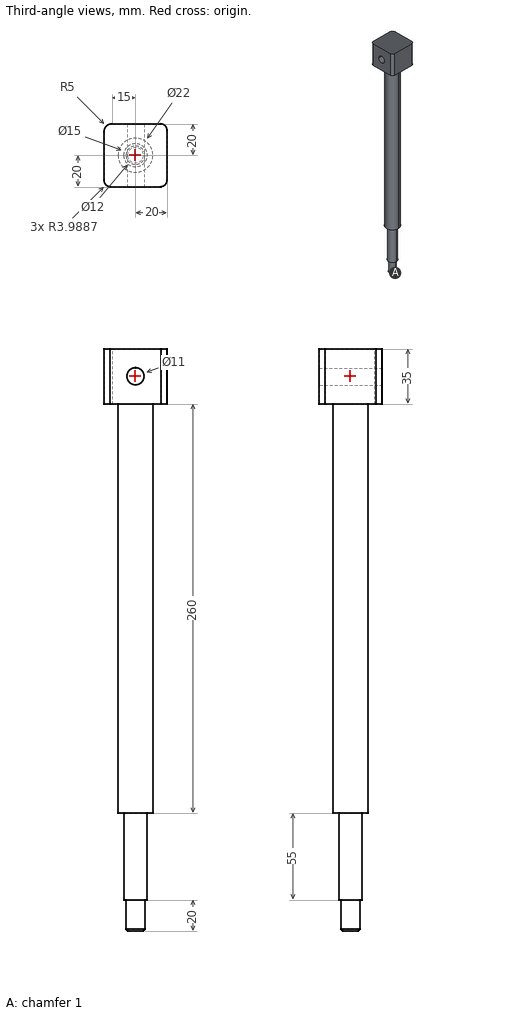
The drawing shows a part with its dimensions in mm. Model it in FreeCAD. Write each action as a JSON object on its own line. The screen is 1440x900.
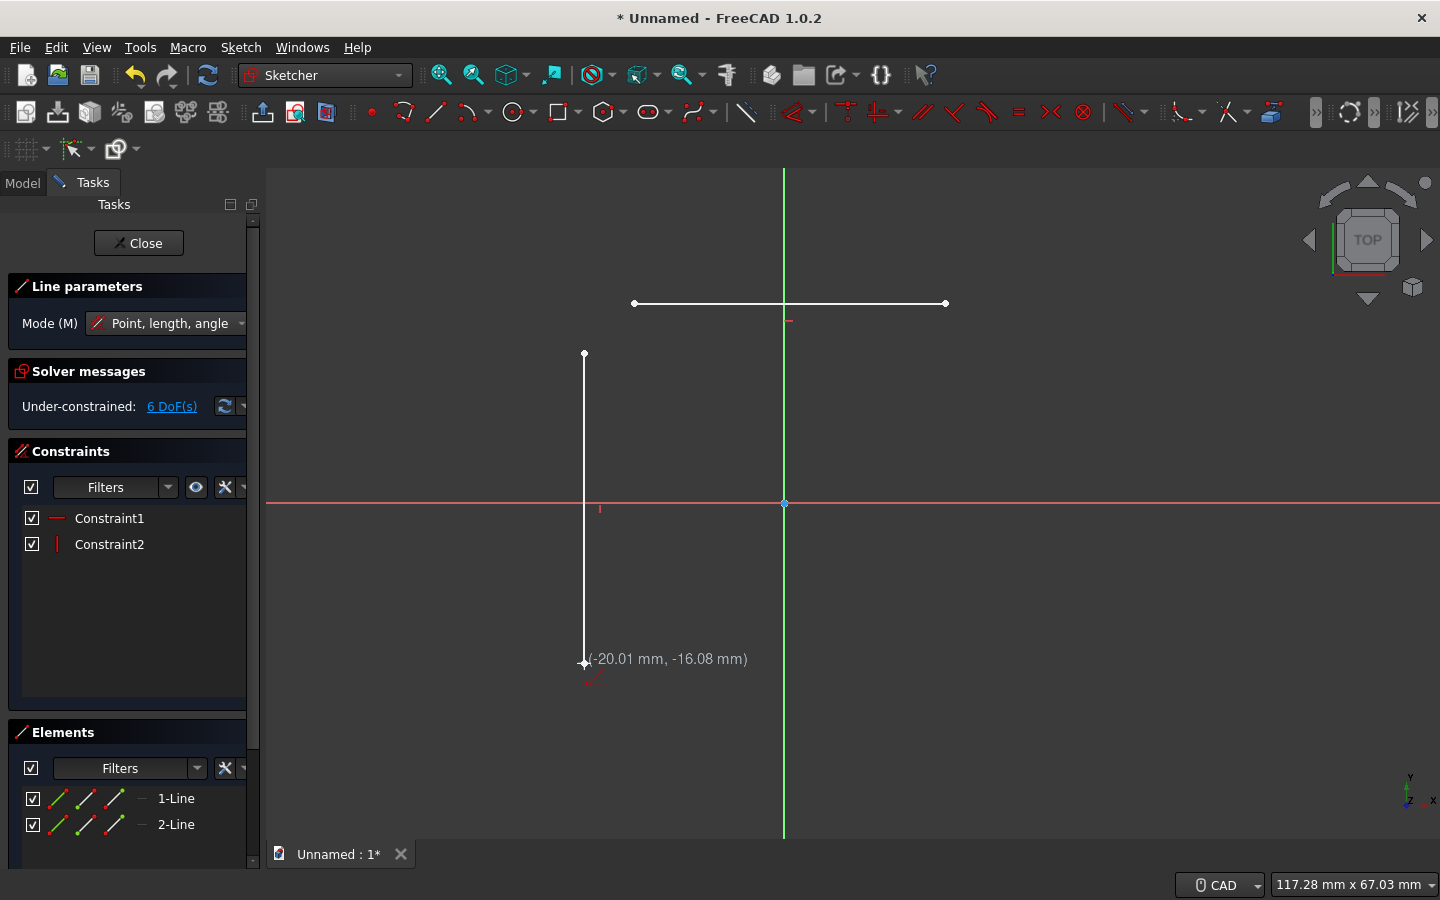
{"action": "left_click", "coordinate": [624, 703]}
{"action": "left_click", "coordinate": [945, 703]}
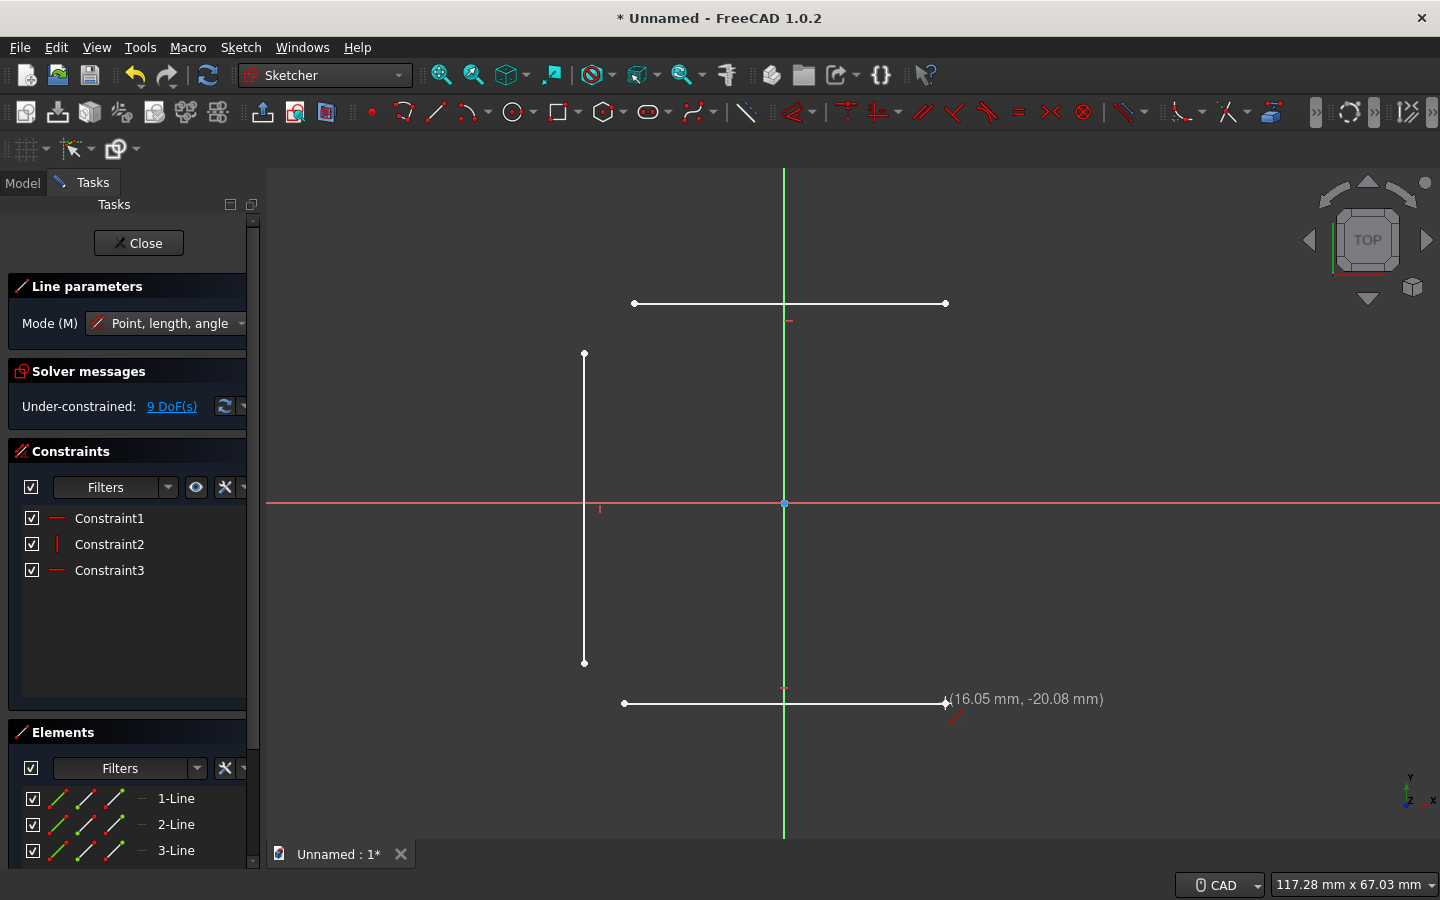
{"action": "left_click", "coordinate": [985, 663]}
{"action": "left_click", "coordinate": [985, 343]}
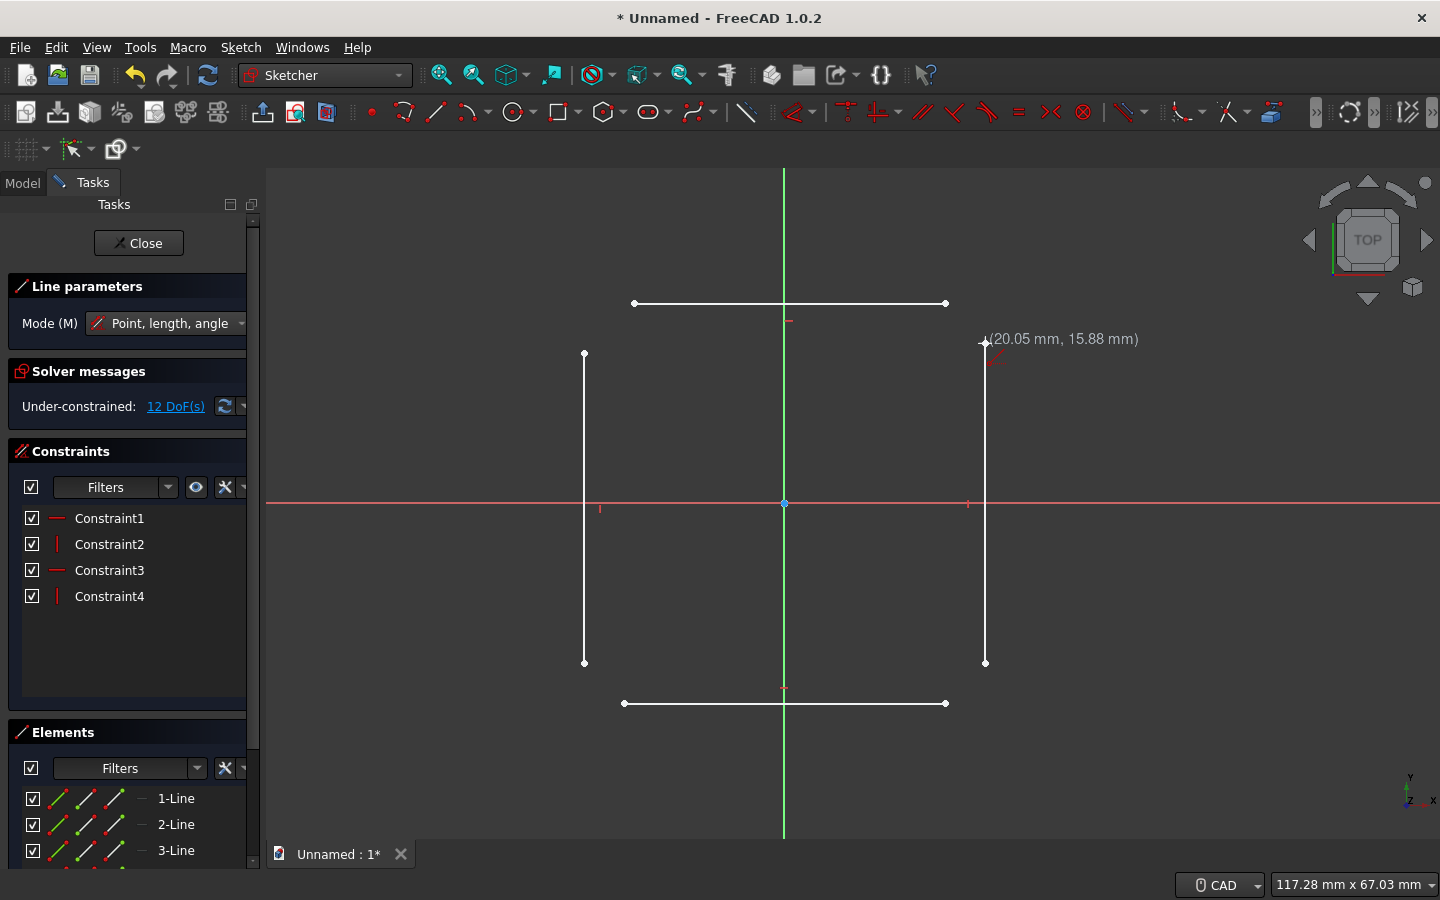
{"action": "left_click", "coordinate": [490, 112]}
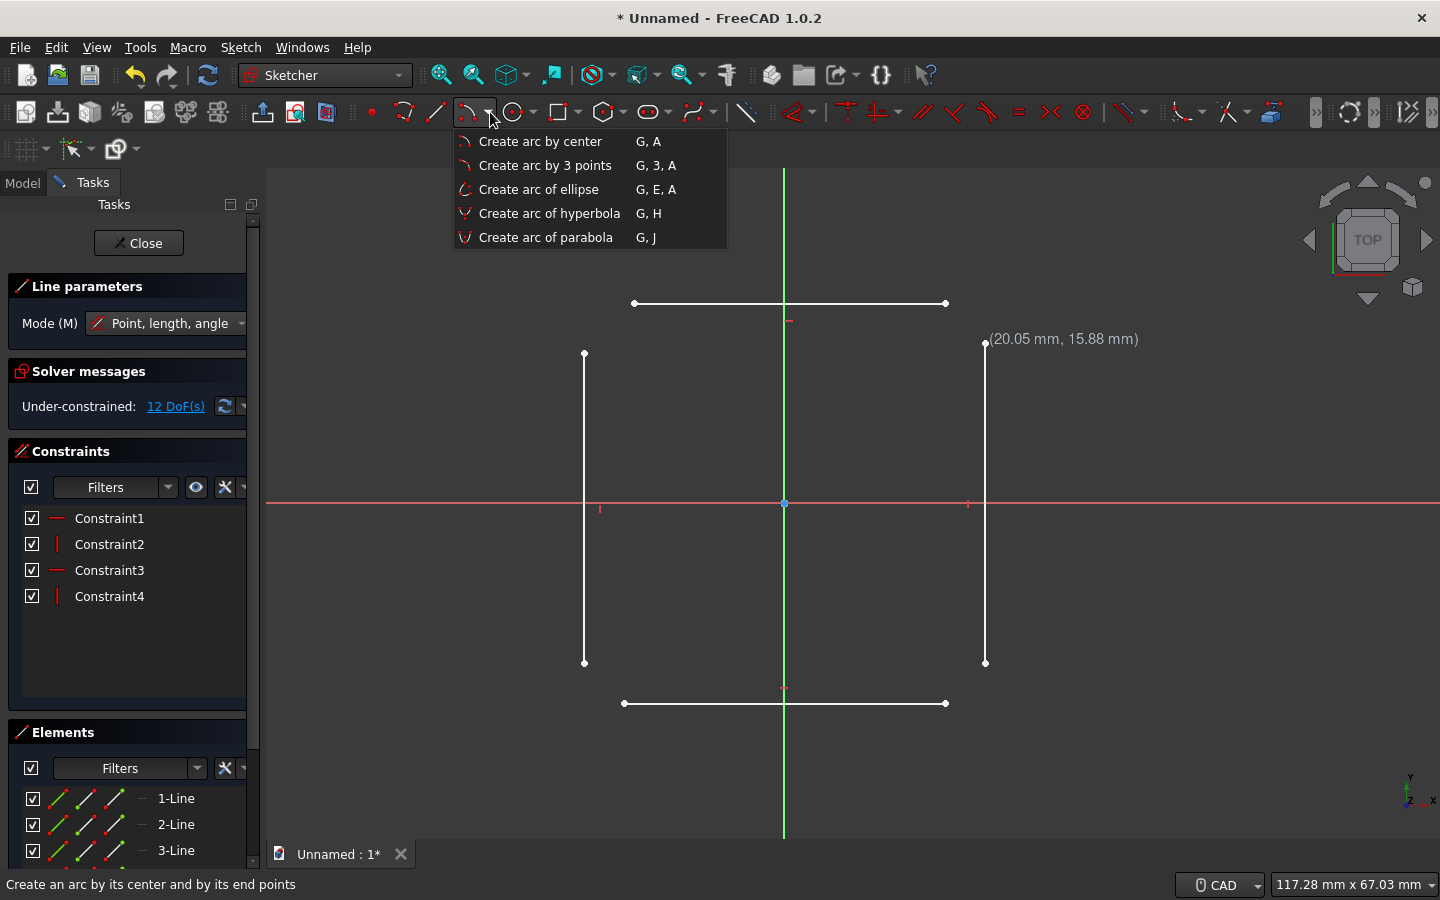
{"action": "left_click", "coordinate": [590, 165]}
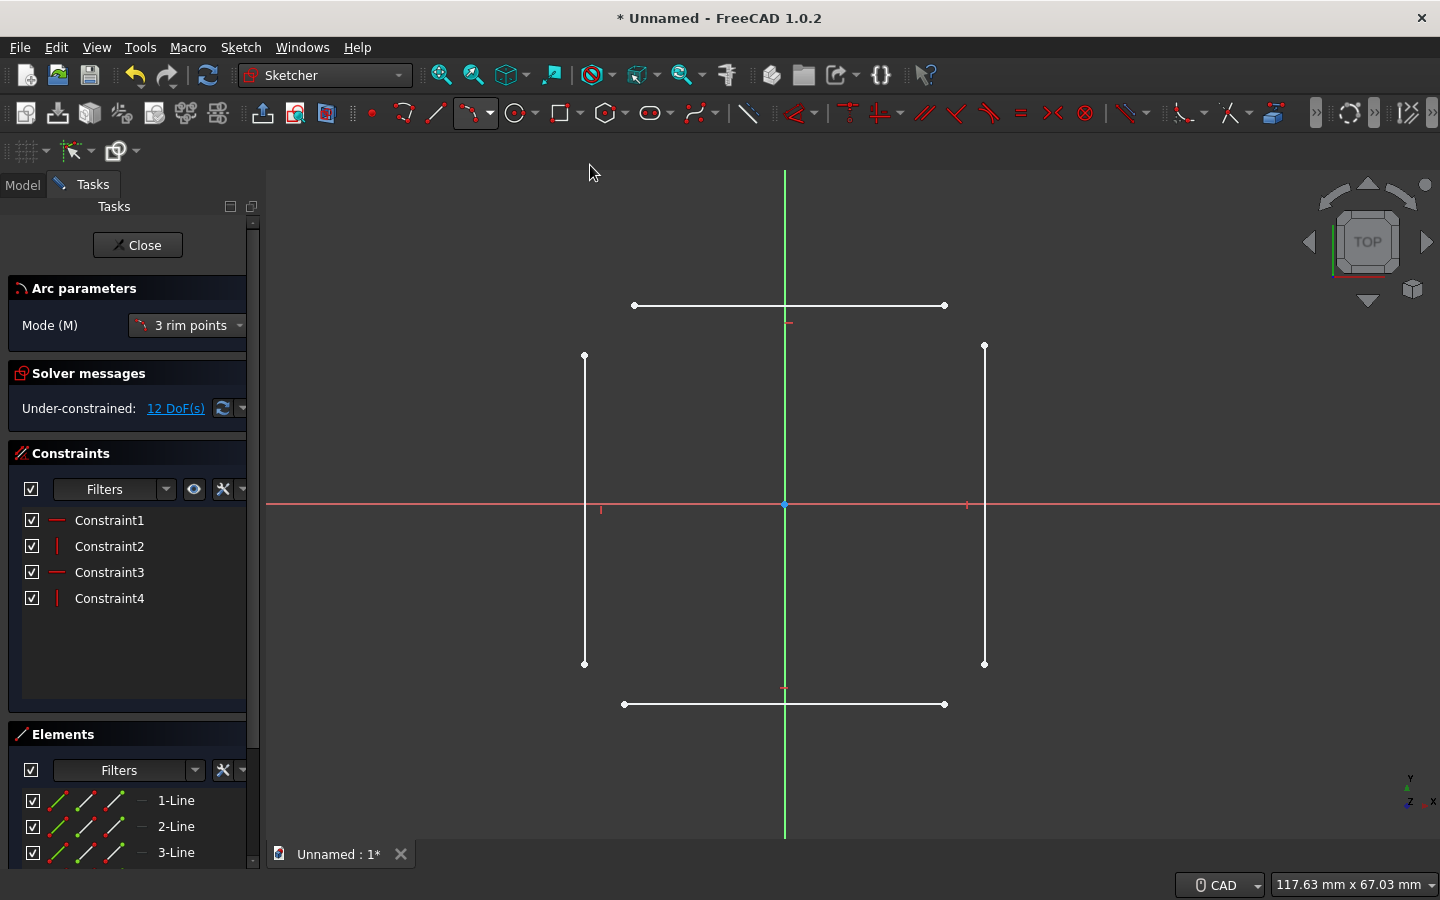
{"action": "left_click", "coordinate": [635, 306]}
{"action": "left_click", "coordinate": [585, 355]}
{"action": "left_click", "coordinate": [600, 319]}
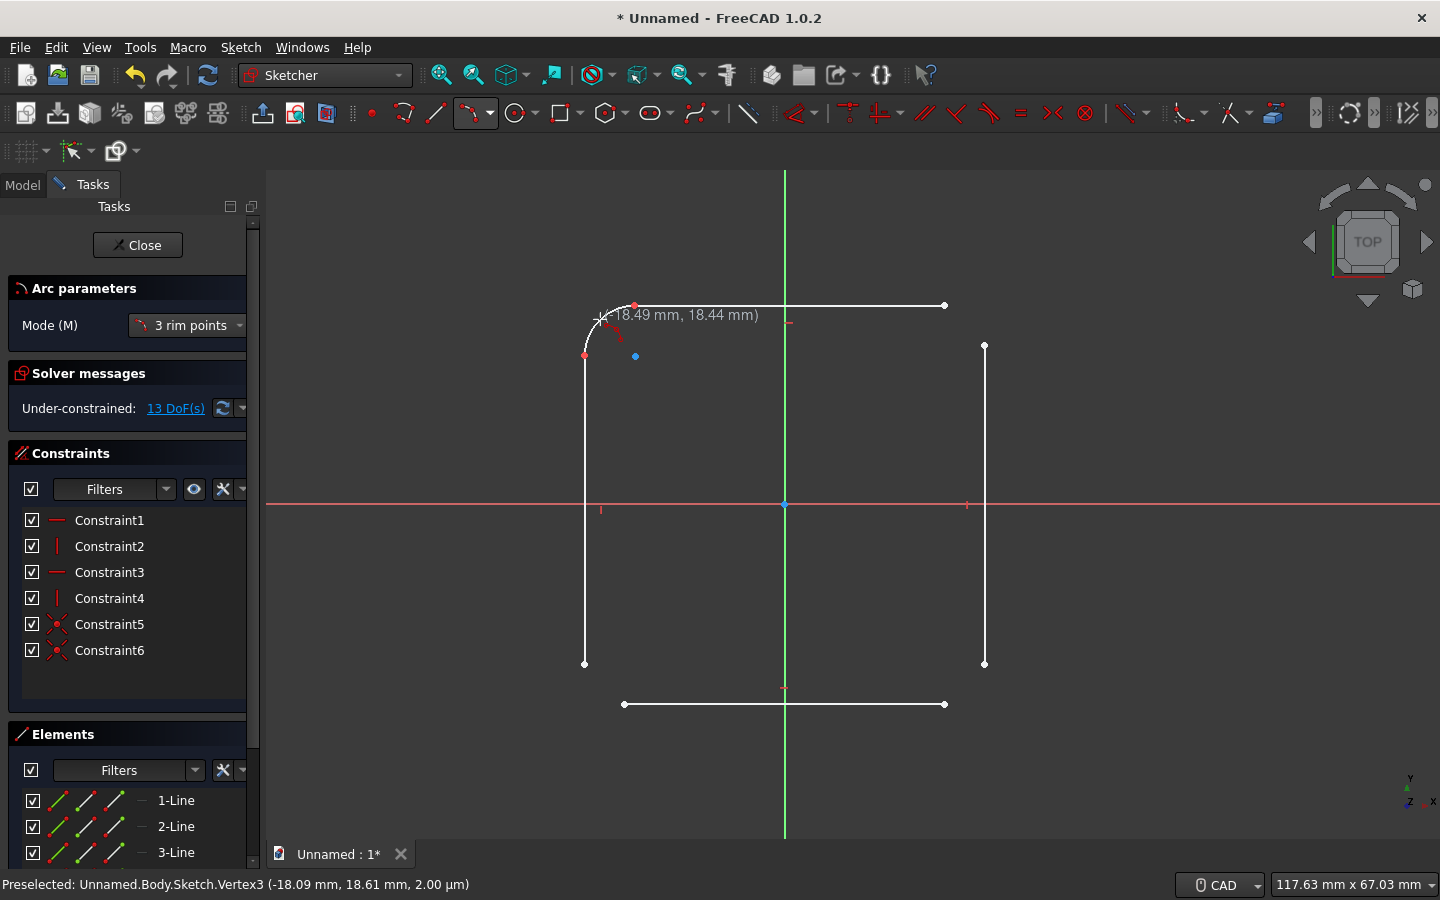
{"action": "left_click", "coordinate": [585, 665]}
{"action": "left_click", "coordinate": [625, 704]}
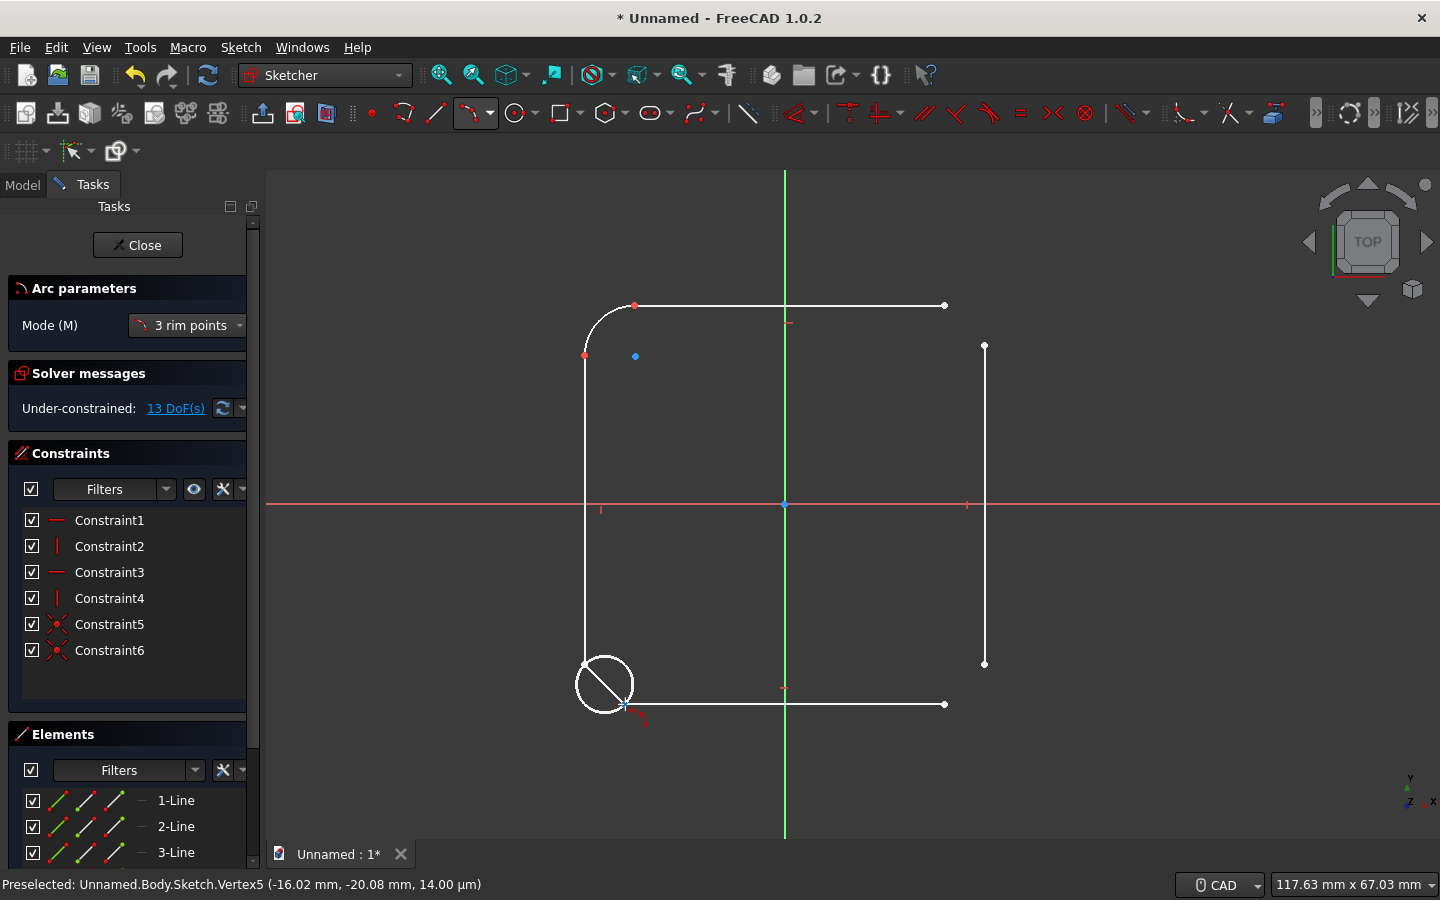
{"action": "scroll", "coordinate": [597, 692], "scroll_direction": "up", "scroll_amount": 2}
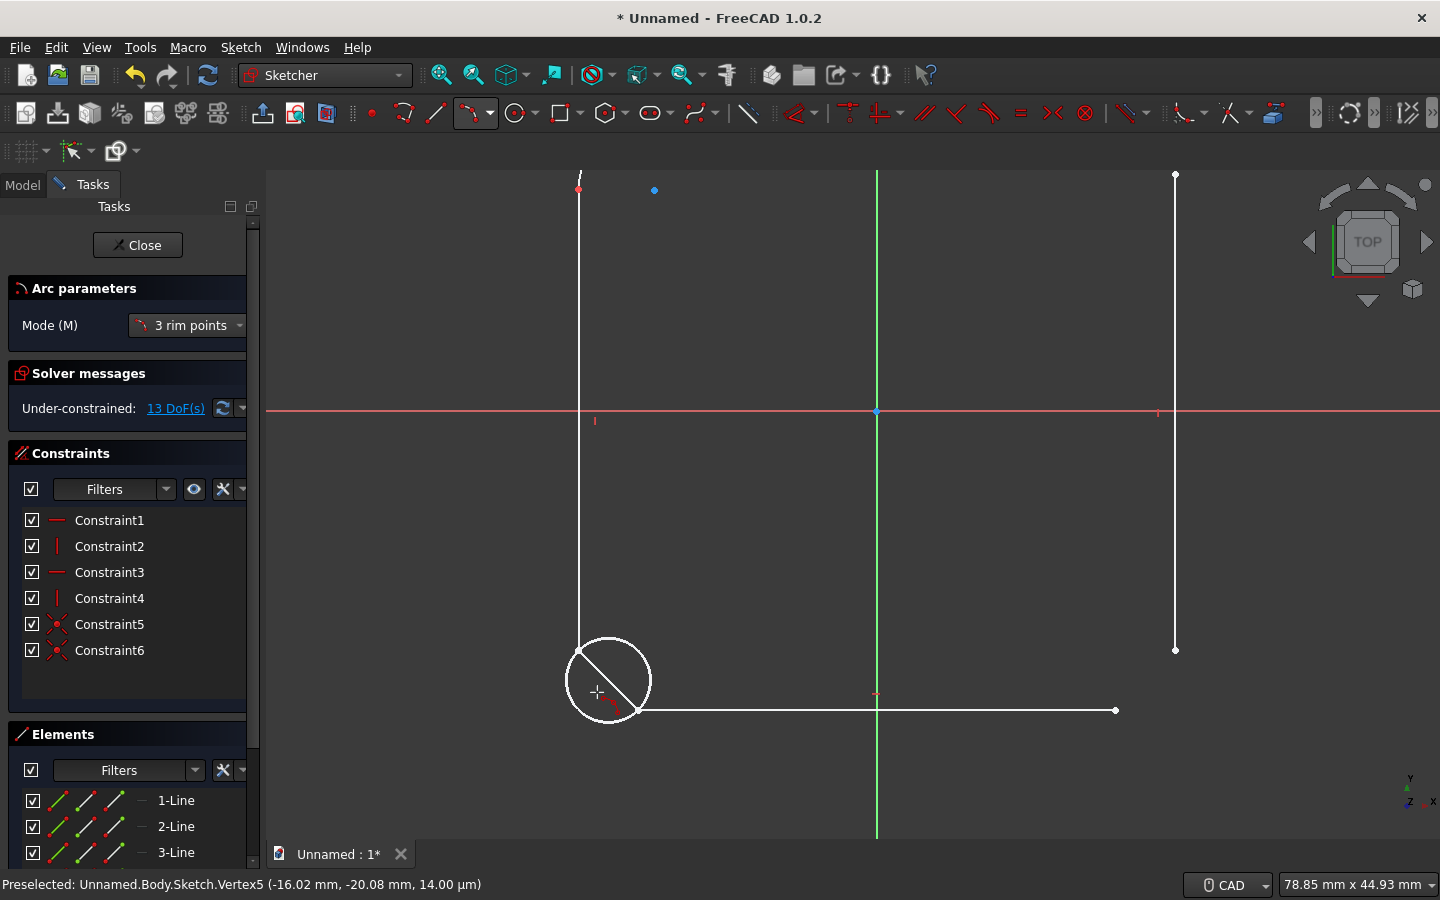
{"action": "left_click", "coordinate": [596, 692]}